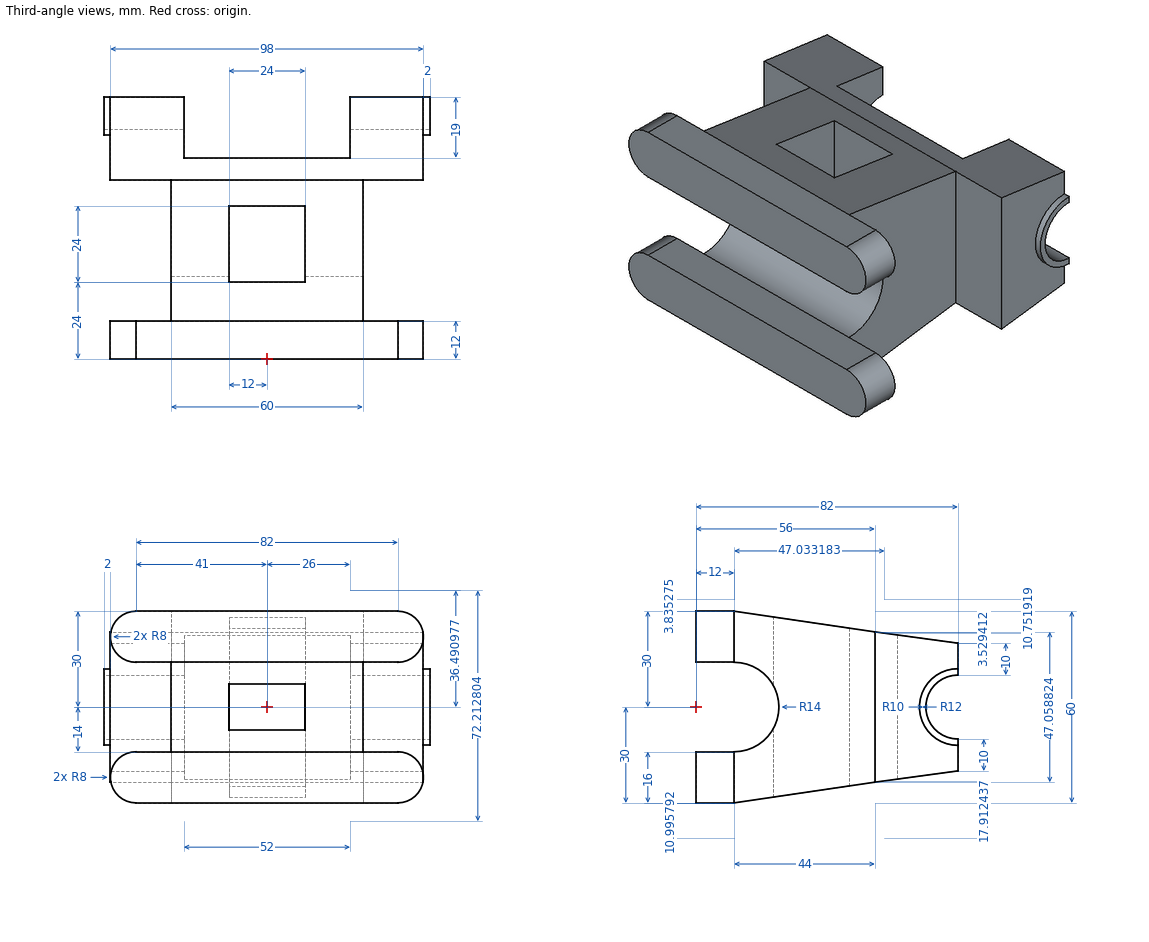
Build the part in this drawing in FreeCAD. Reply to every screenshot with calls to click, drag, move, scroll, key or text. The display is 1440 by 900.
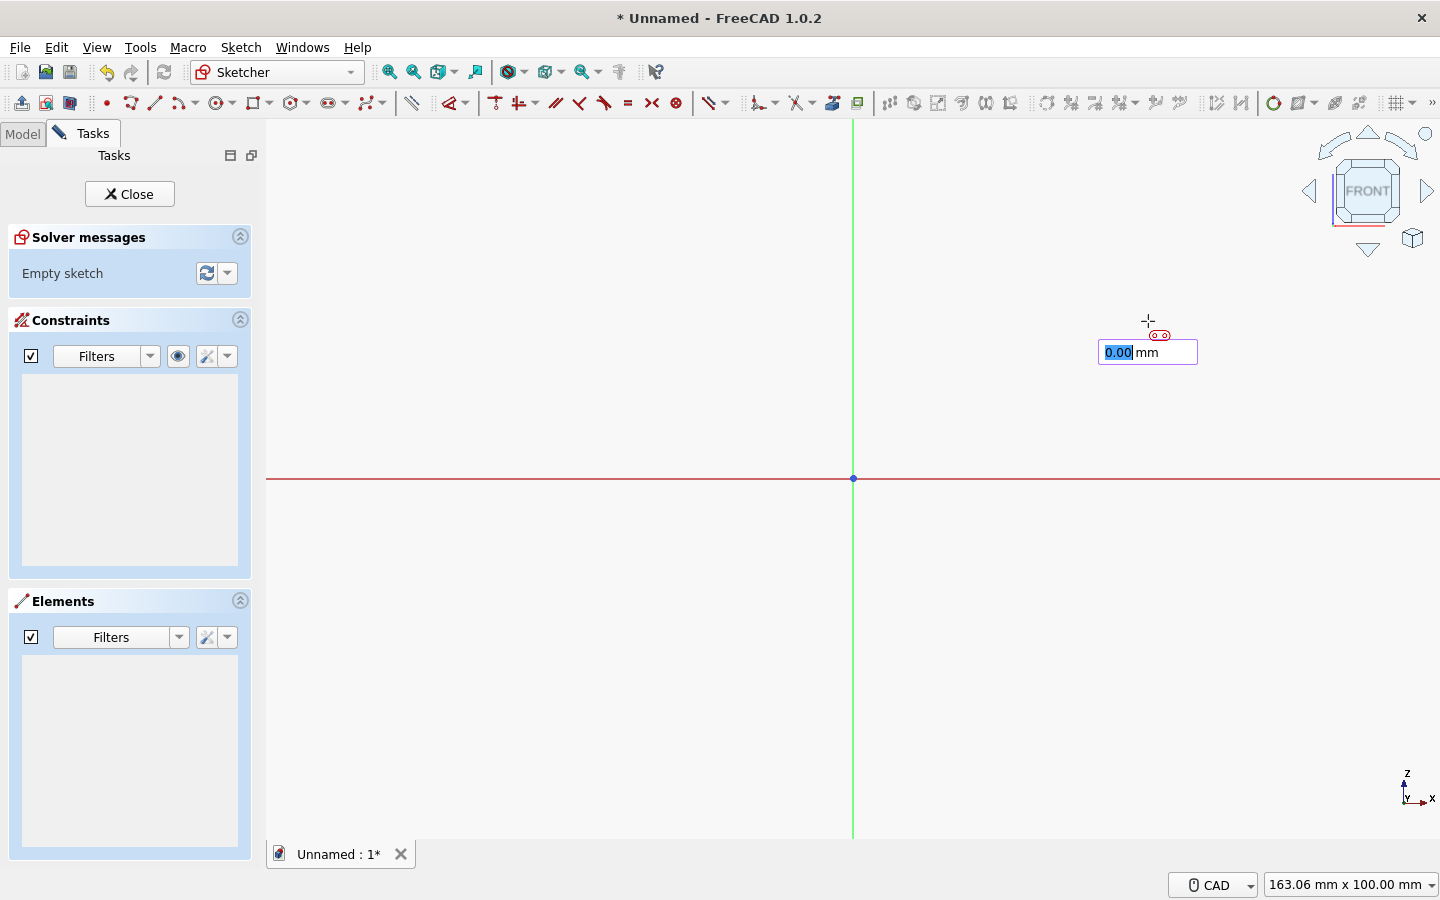
click(942, 378)
key(Escape)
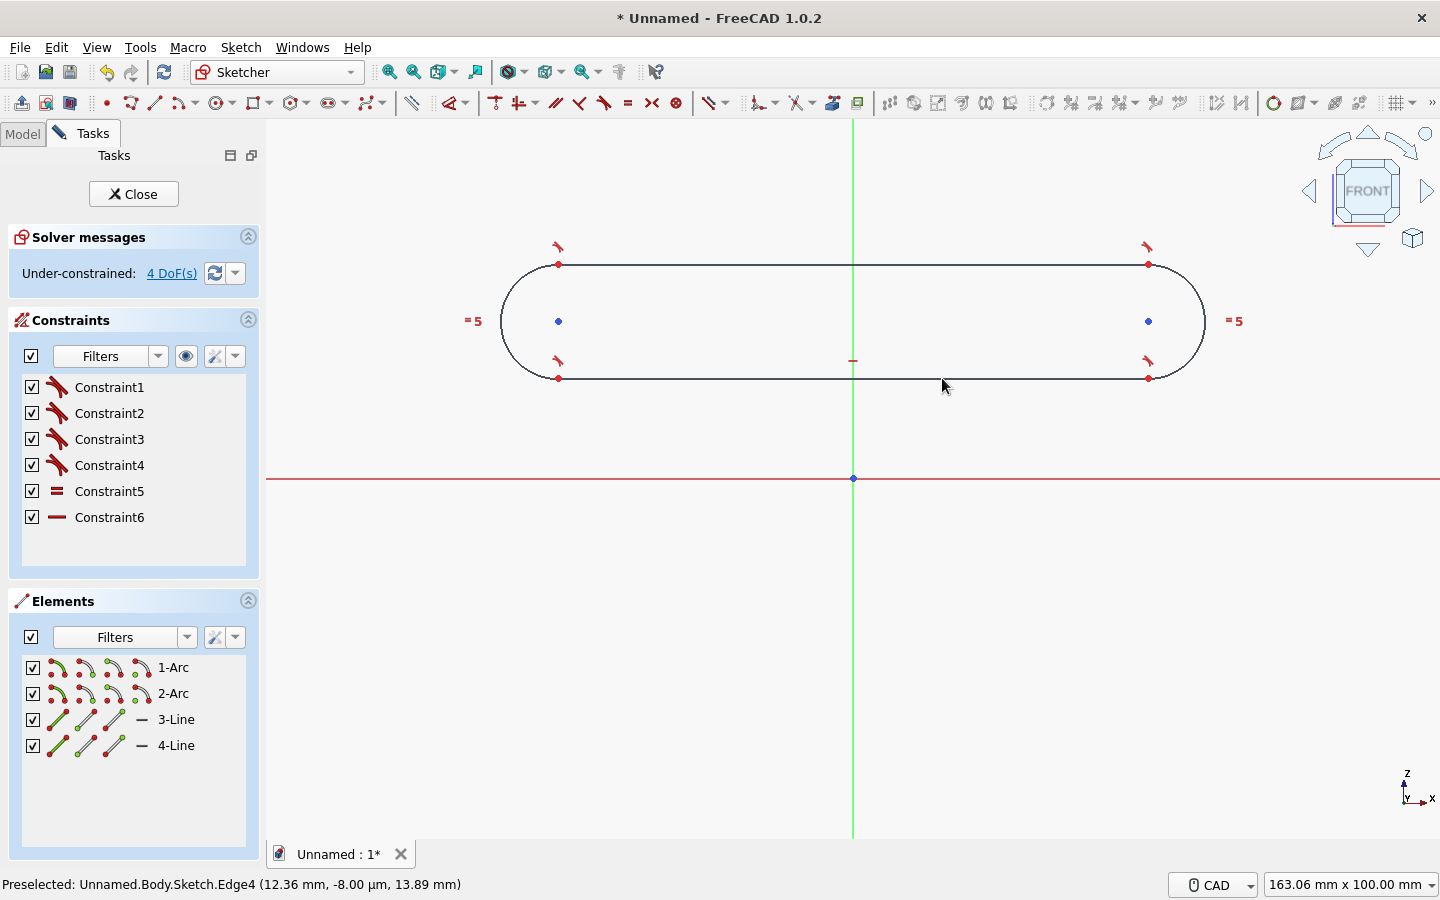
click(450, 104)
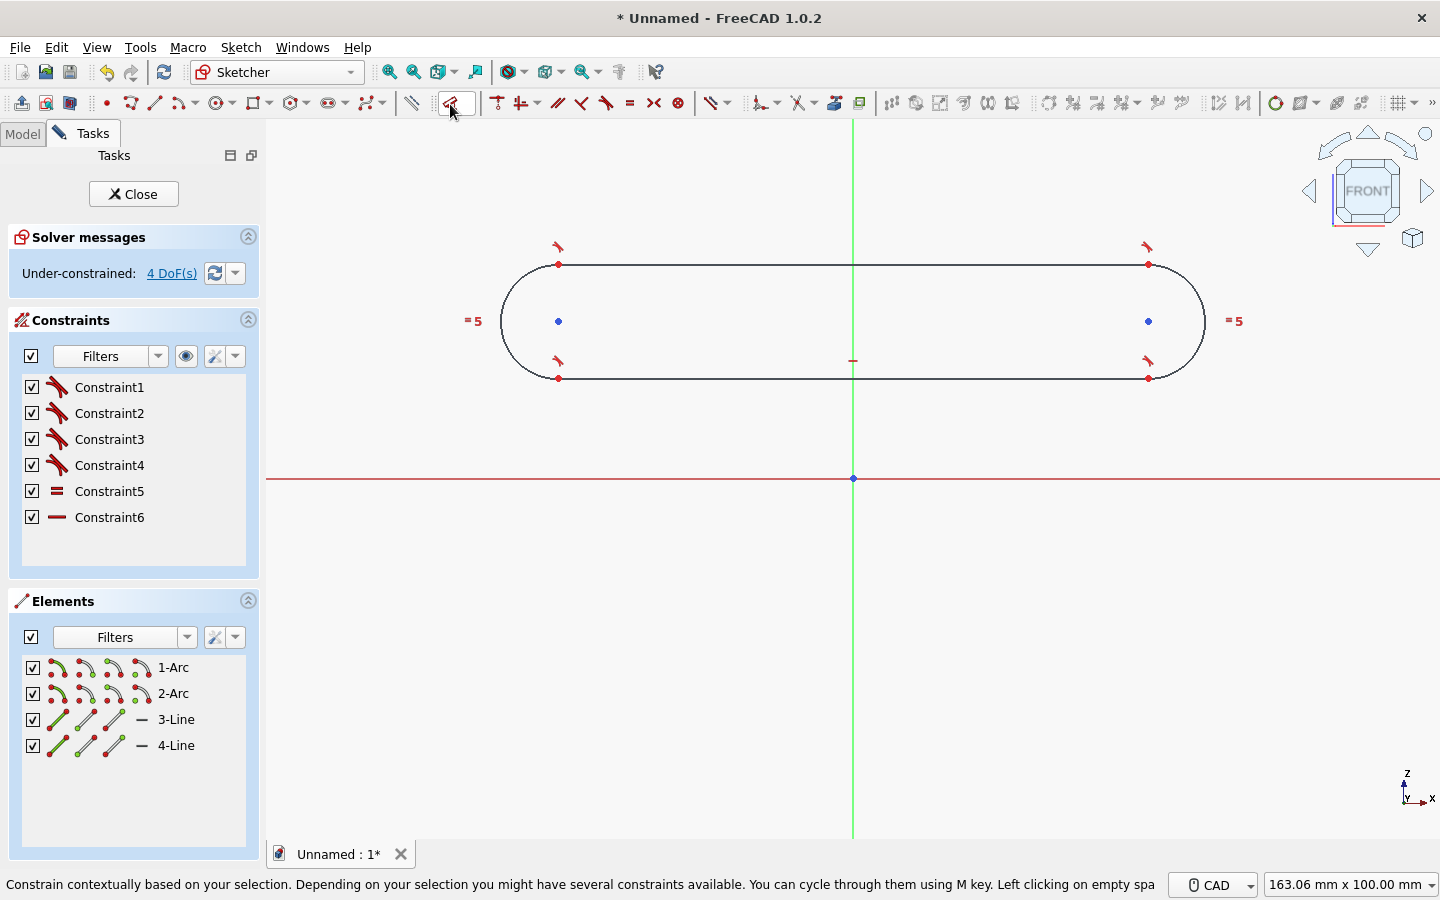
click(512, 288)
click(486, 269)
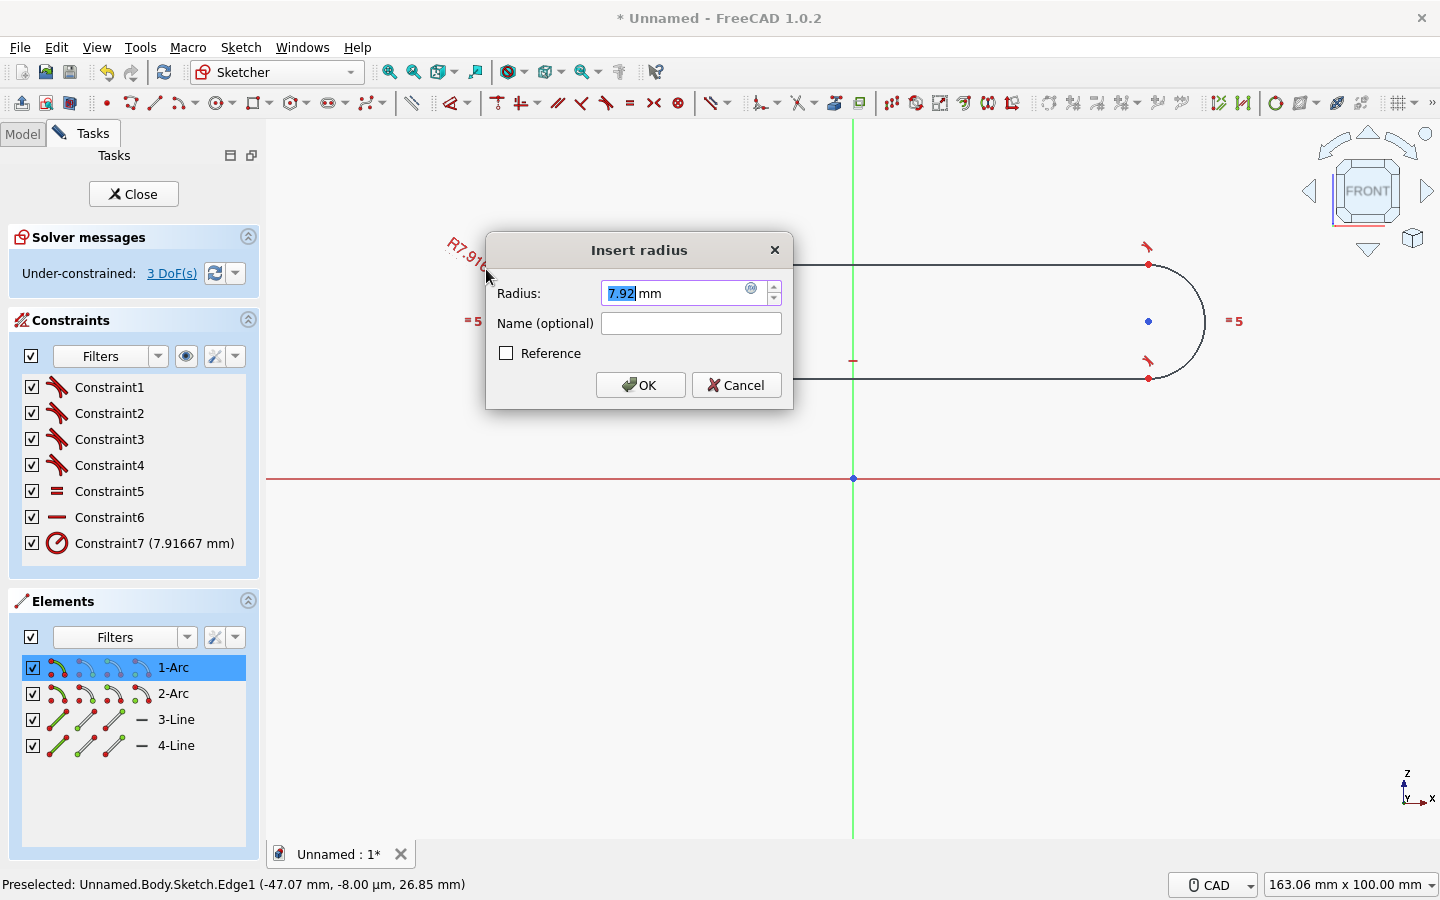
text(8)
key(Return)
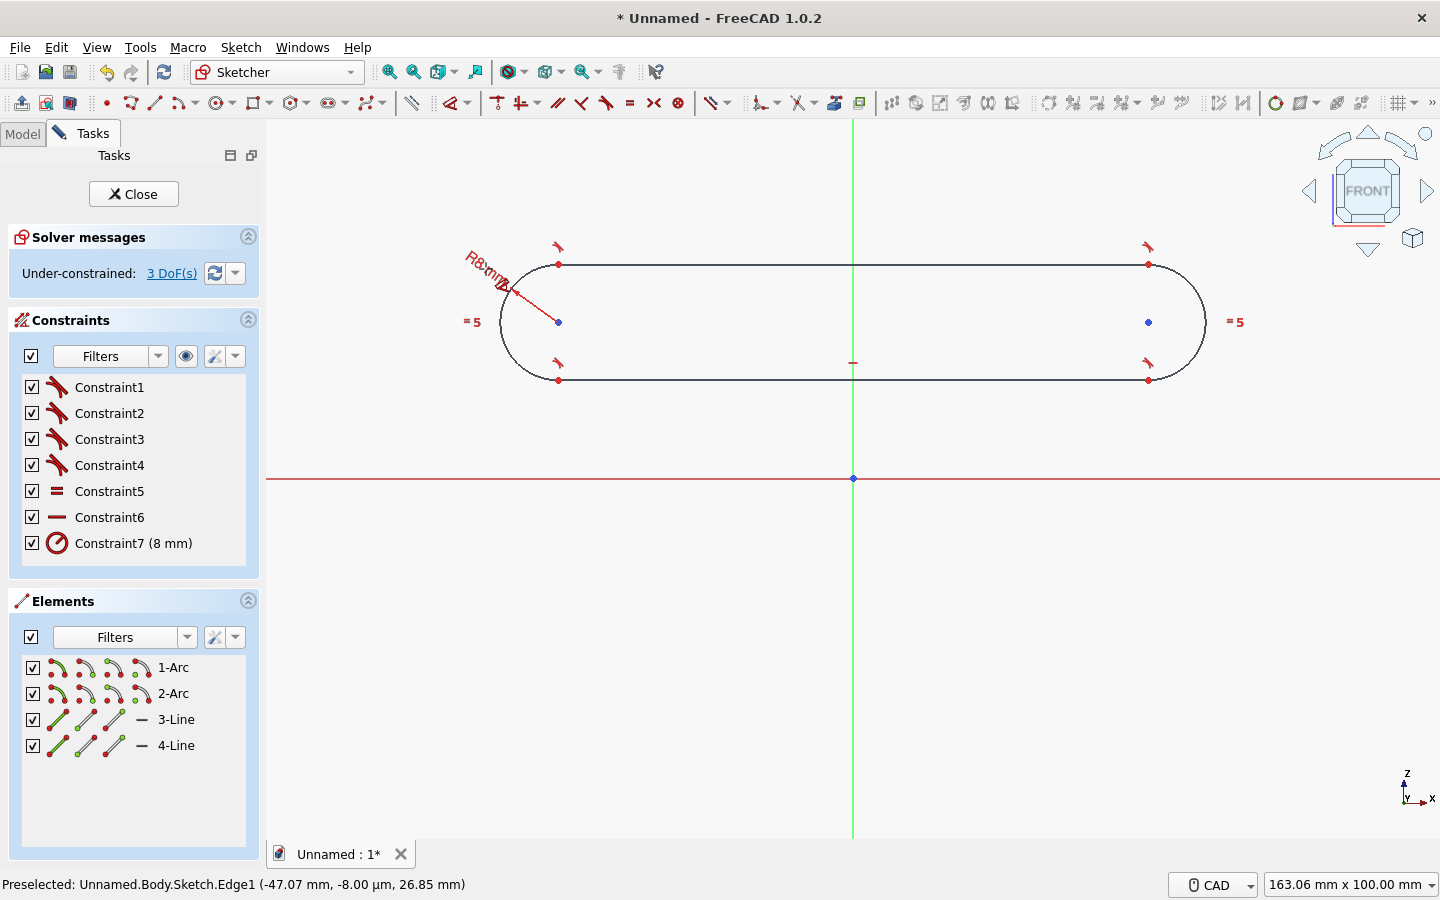
click(735, 265)
click(717, 231)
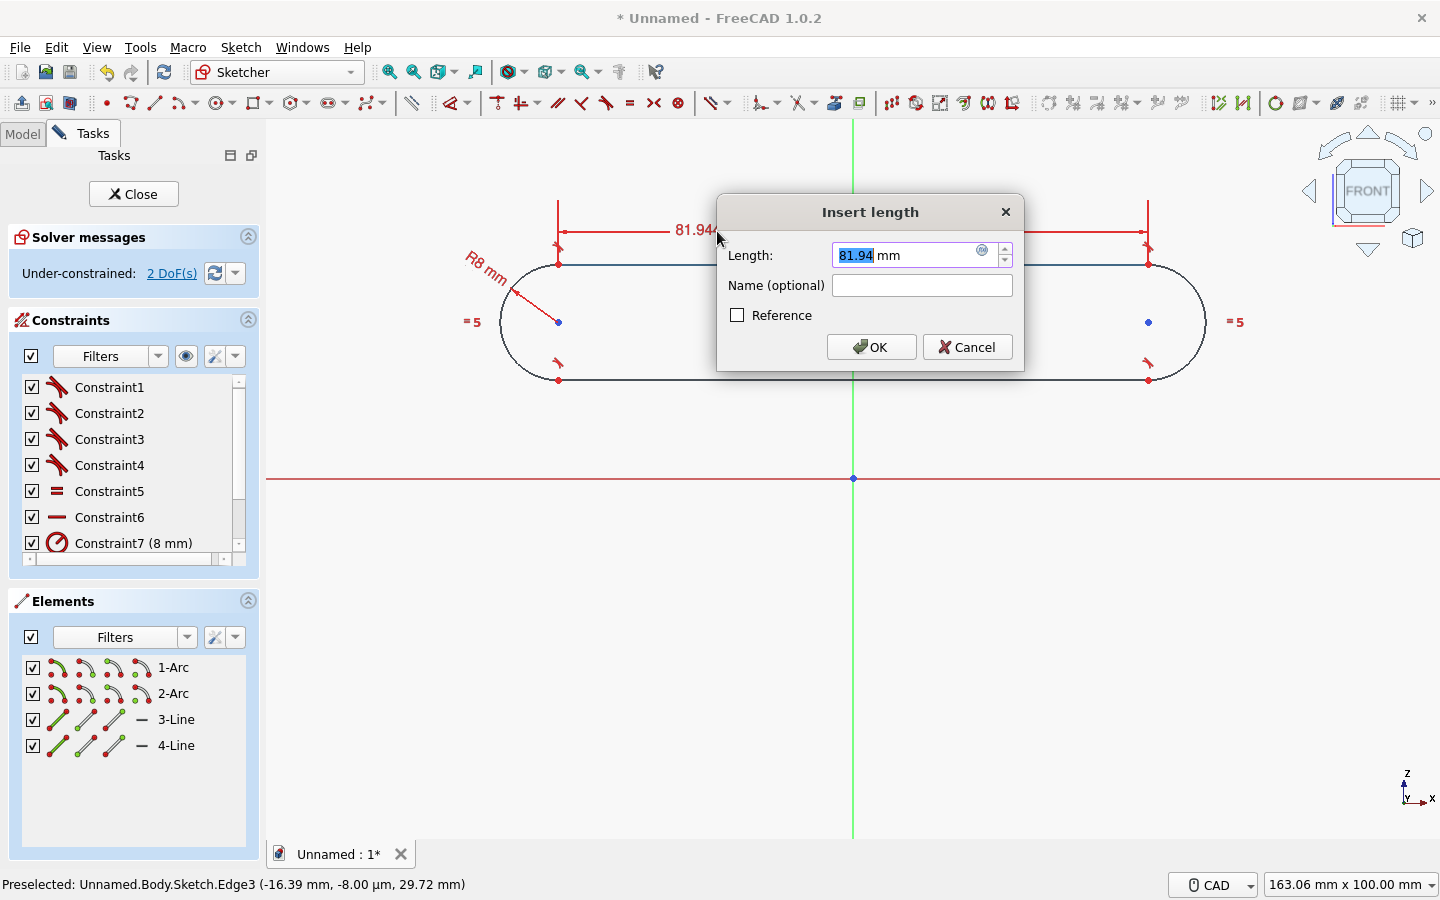
text(82)
key(Return)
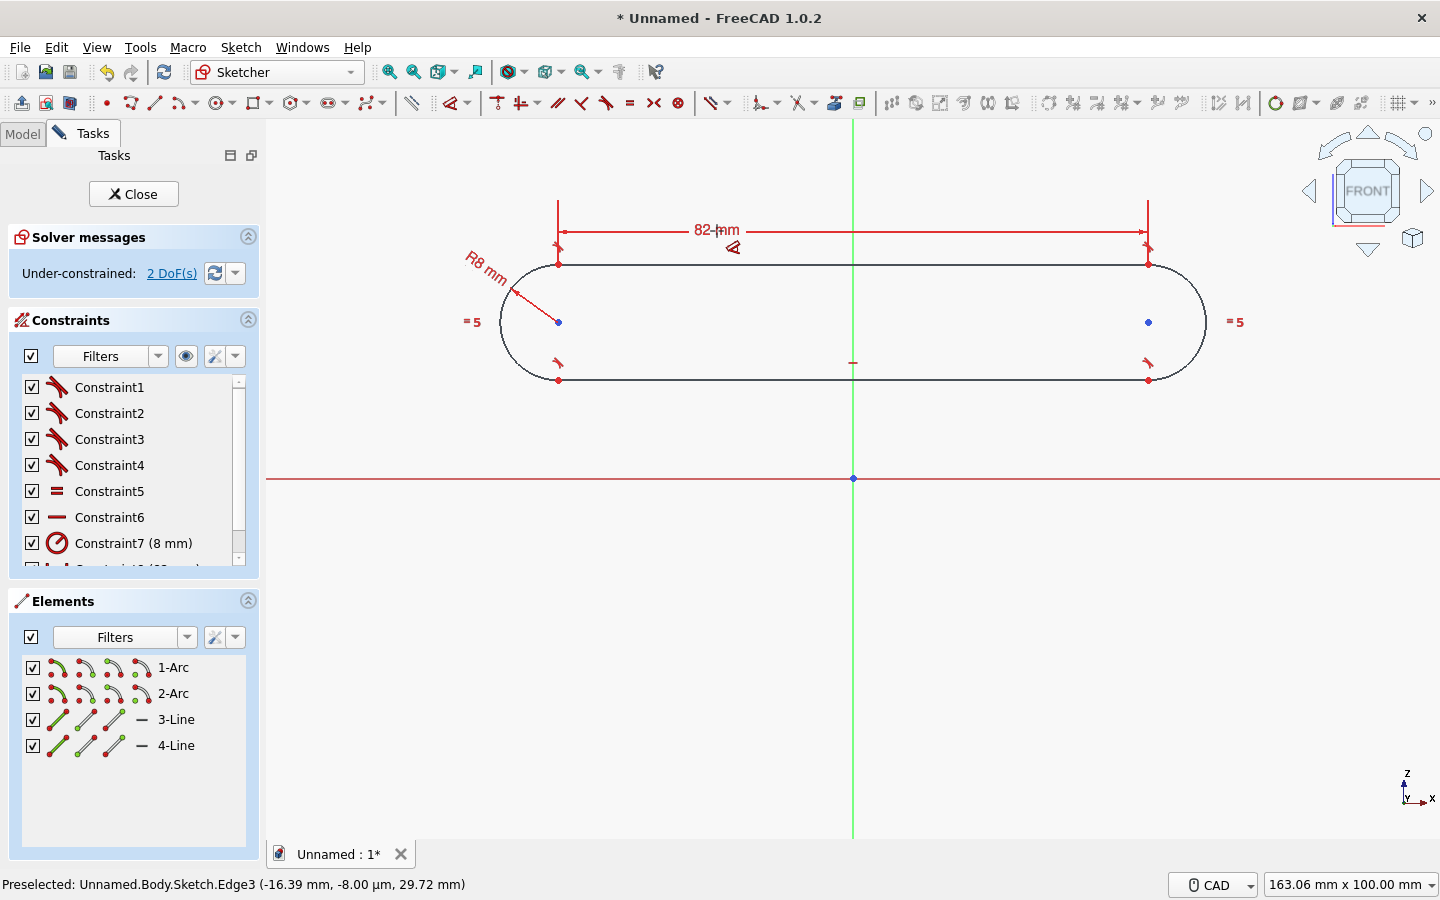
click(558, 265)
click(706, 513)